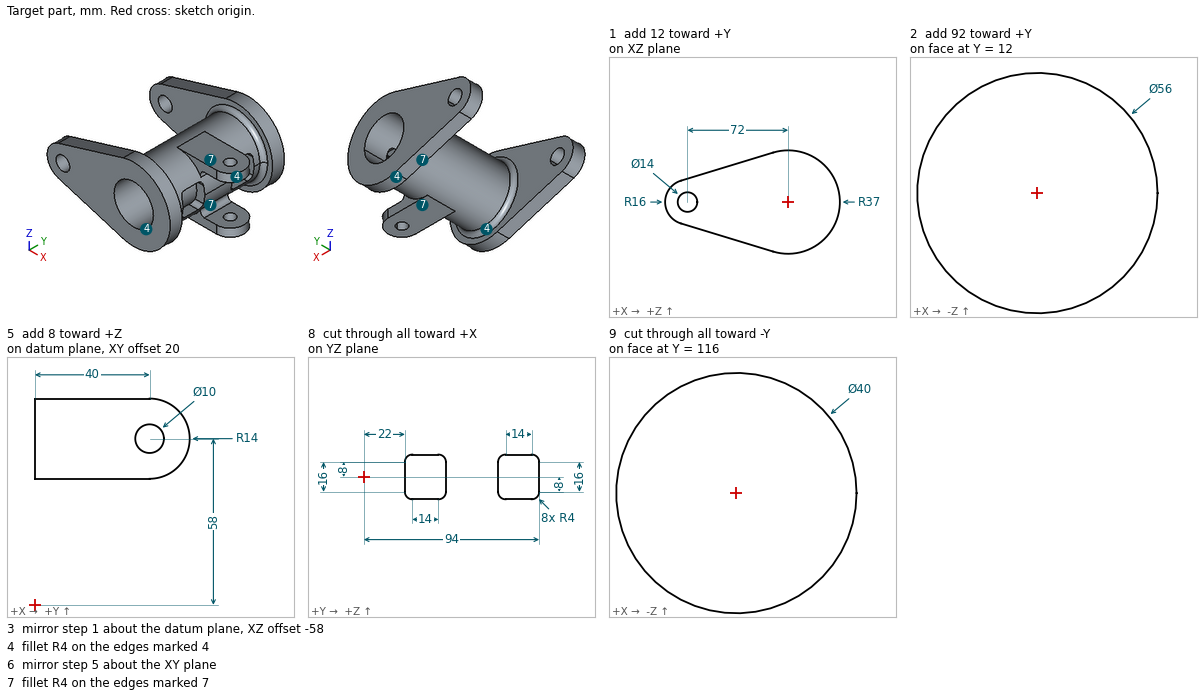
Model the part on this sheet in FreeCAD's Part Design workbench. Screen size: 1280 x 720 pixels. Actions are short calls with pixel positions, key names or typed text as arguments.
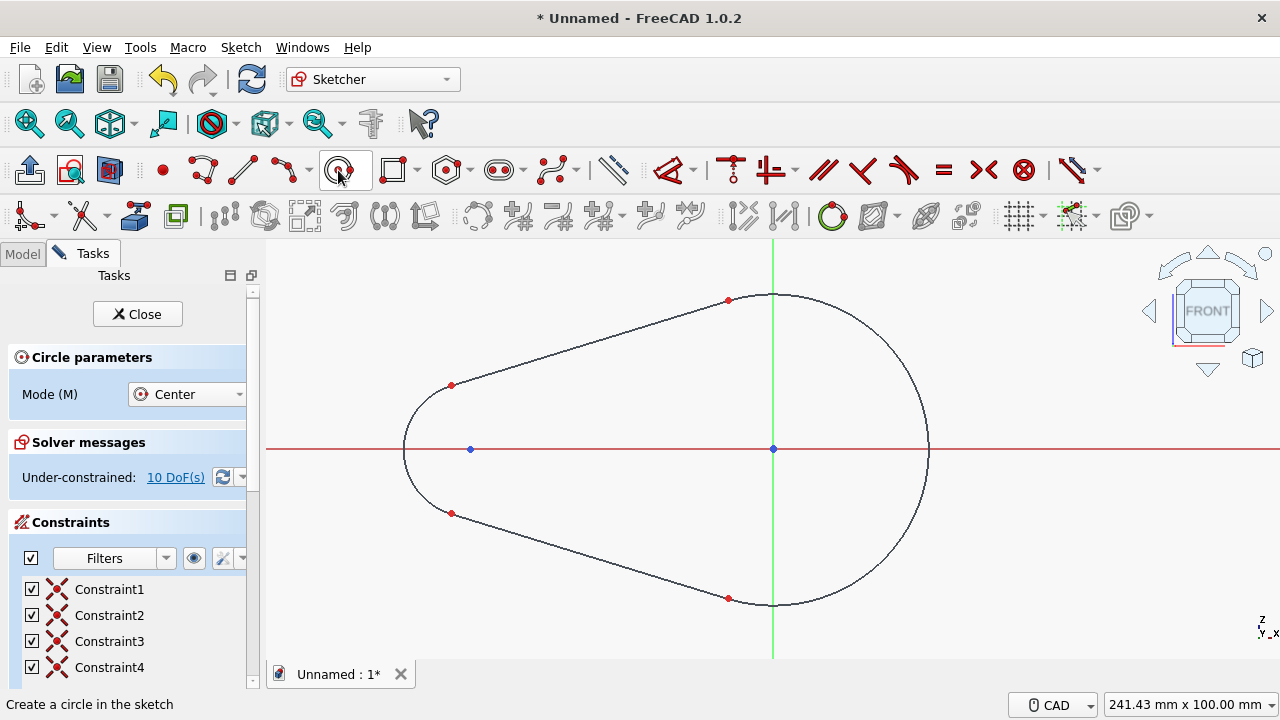
click(471, 449)
move(491, 428)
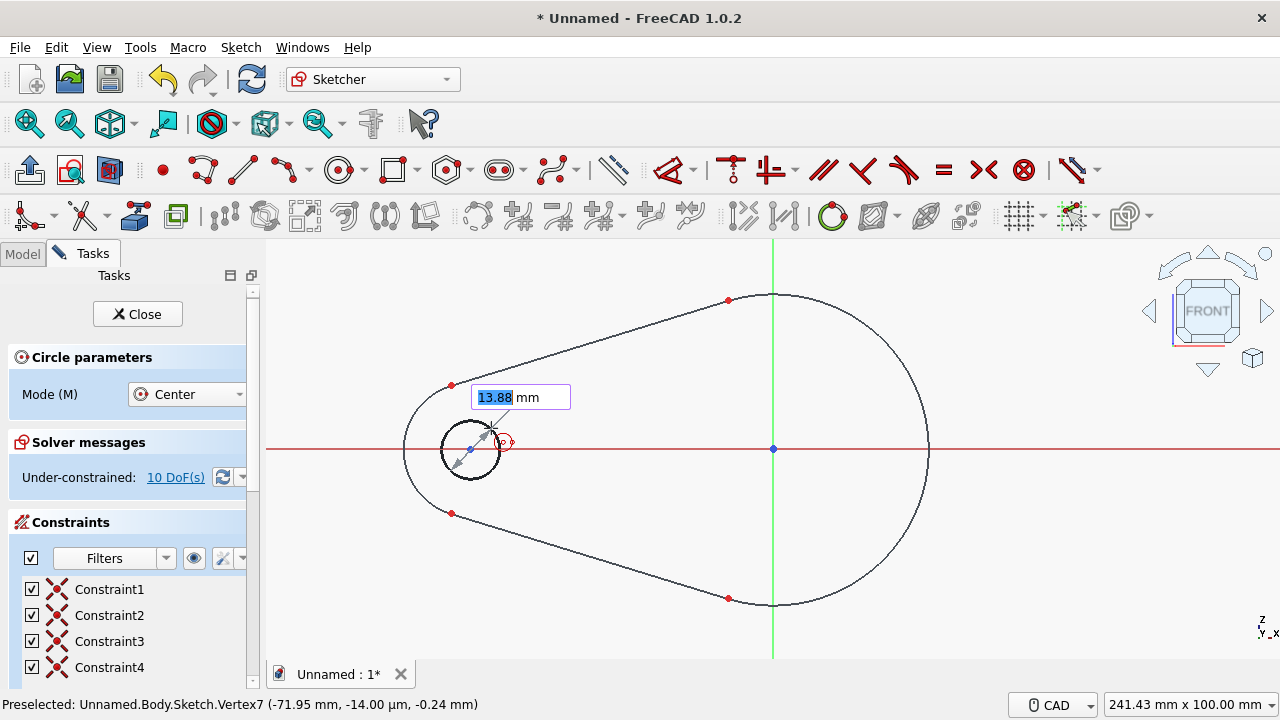
text(14)
key(Return)
key(Escape)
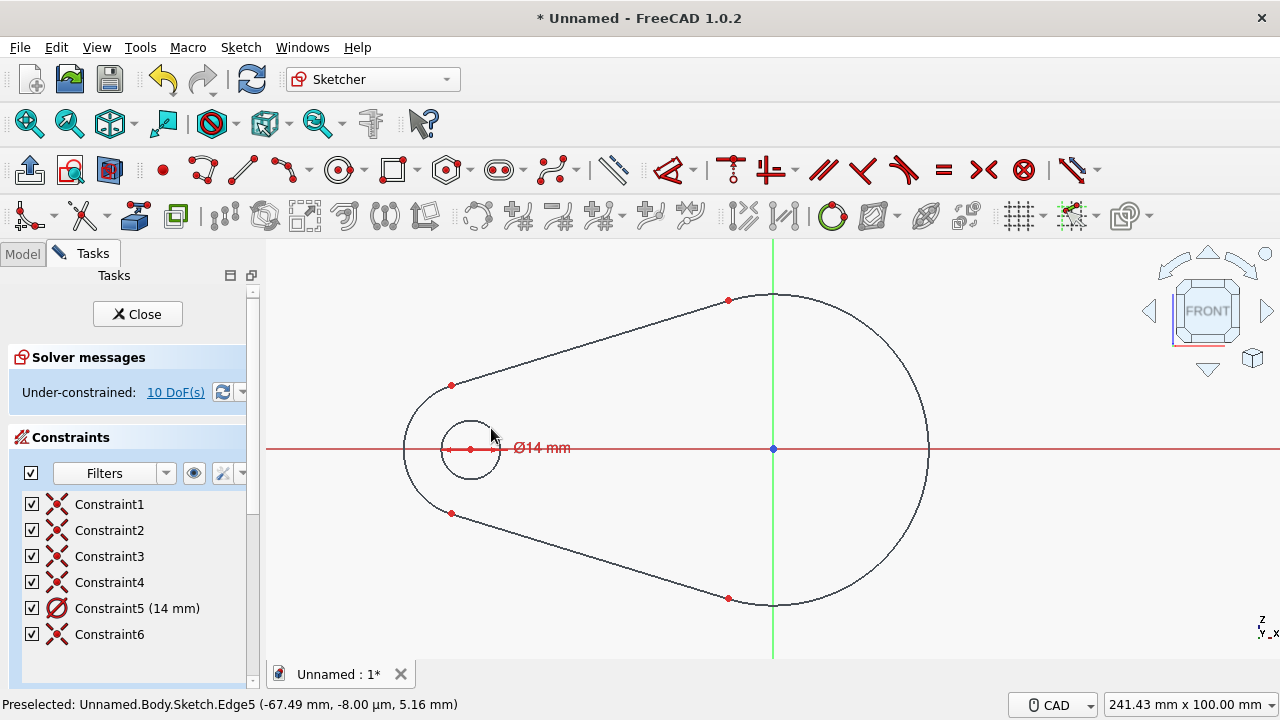
click(645, 574)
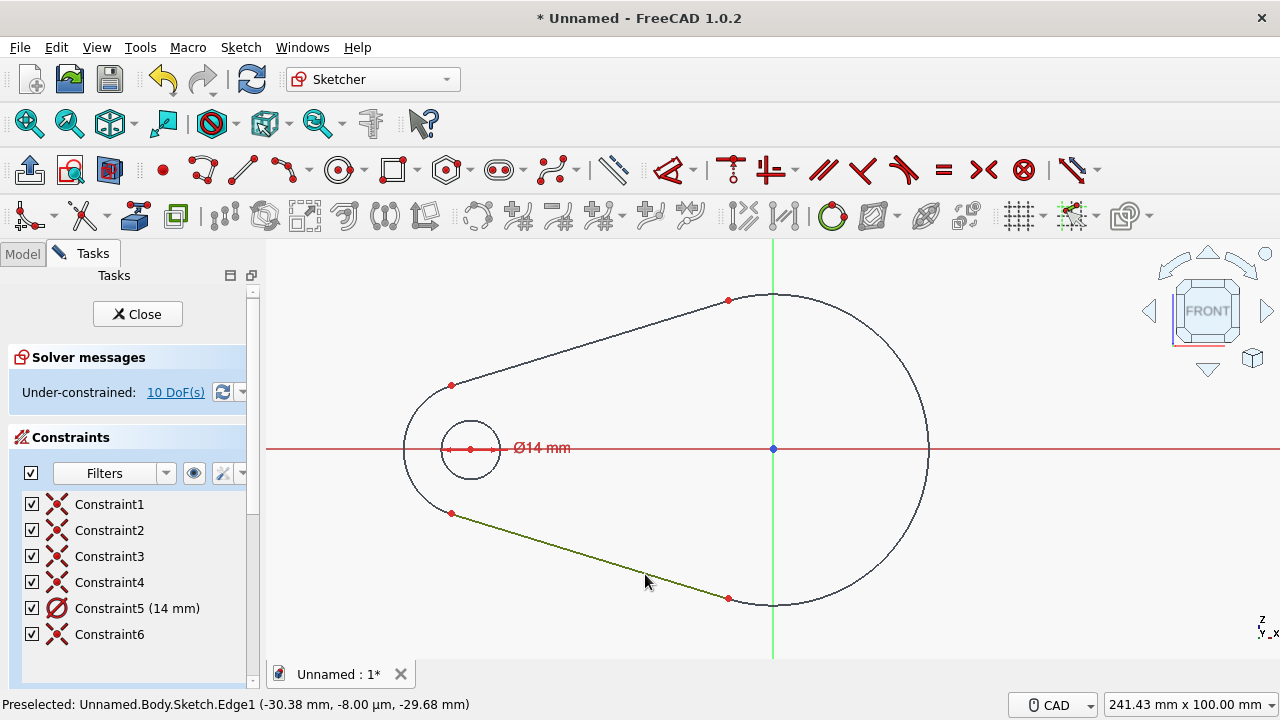
click(412, 417)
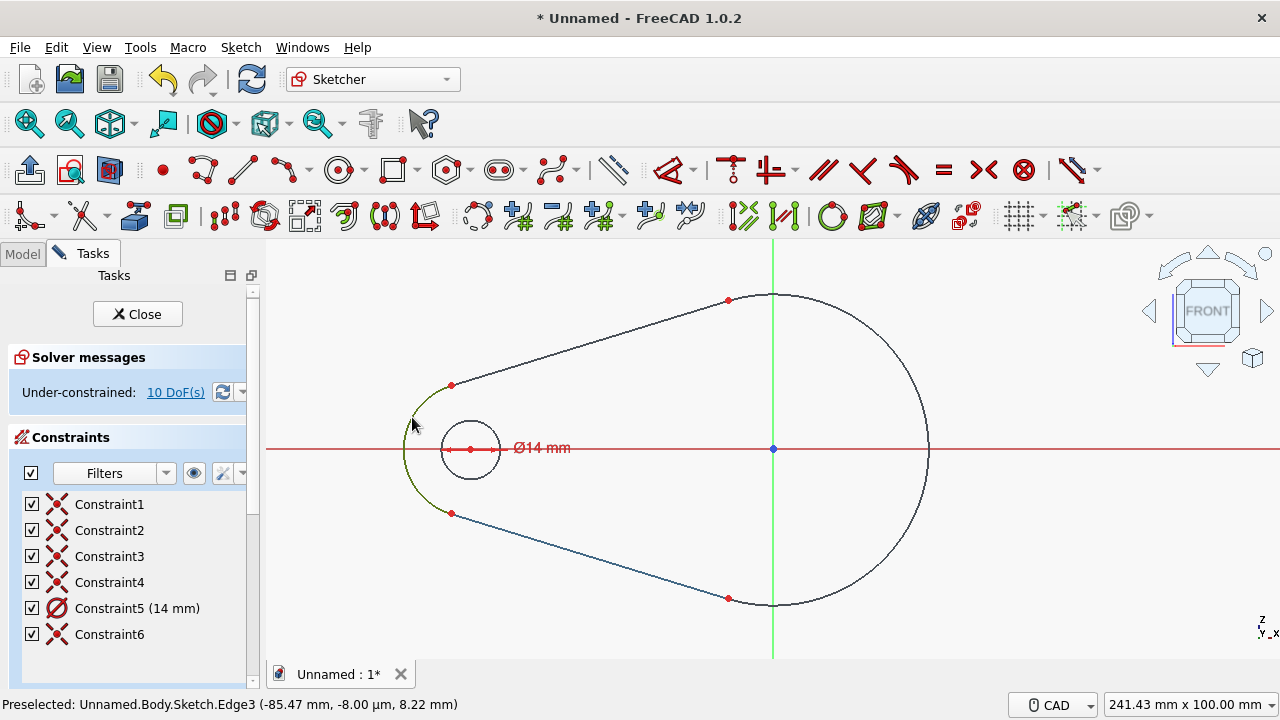
click(904, 170)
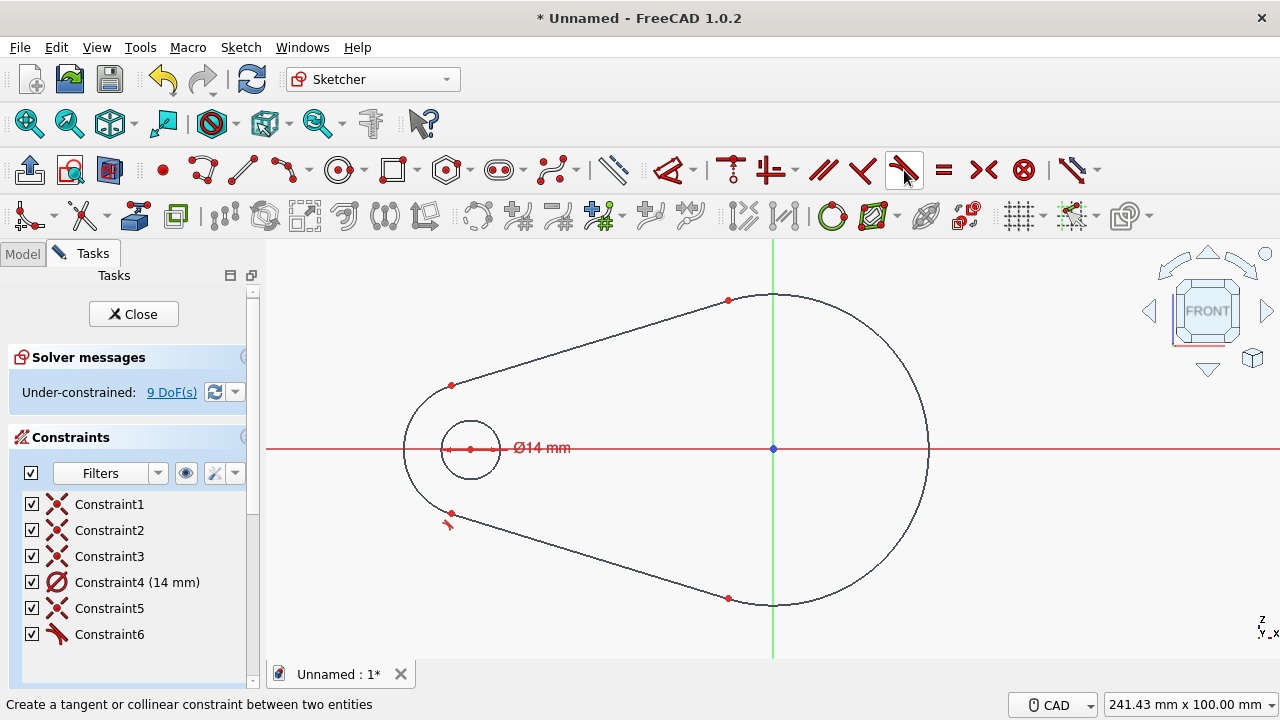
click(645, 574)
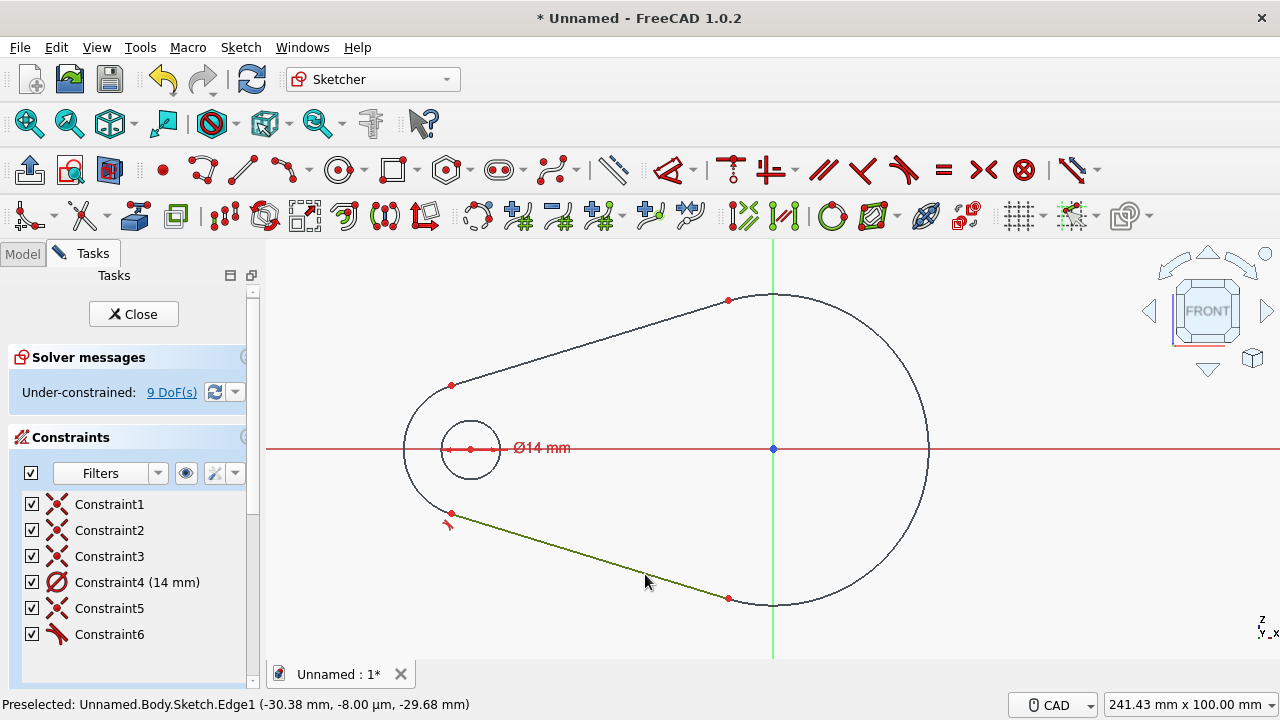
click(887, 556)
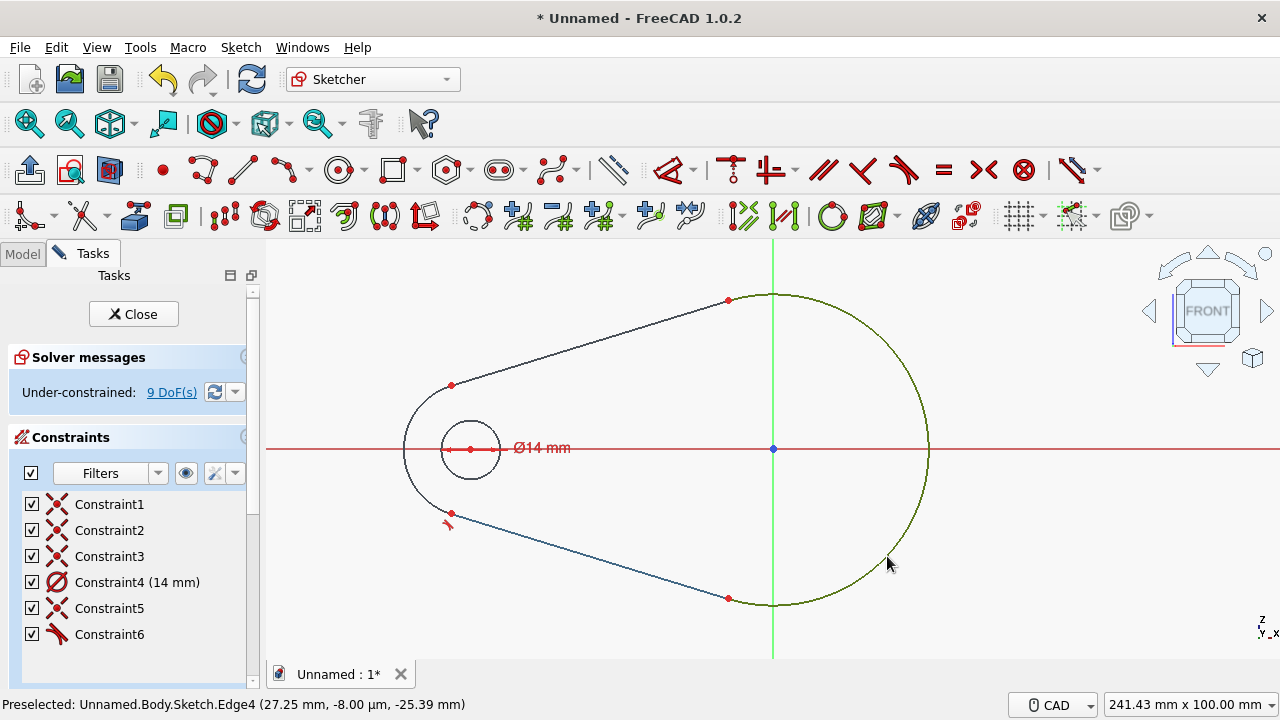
click(904, 170)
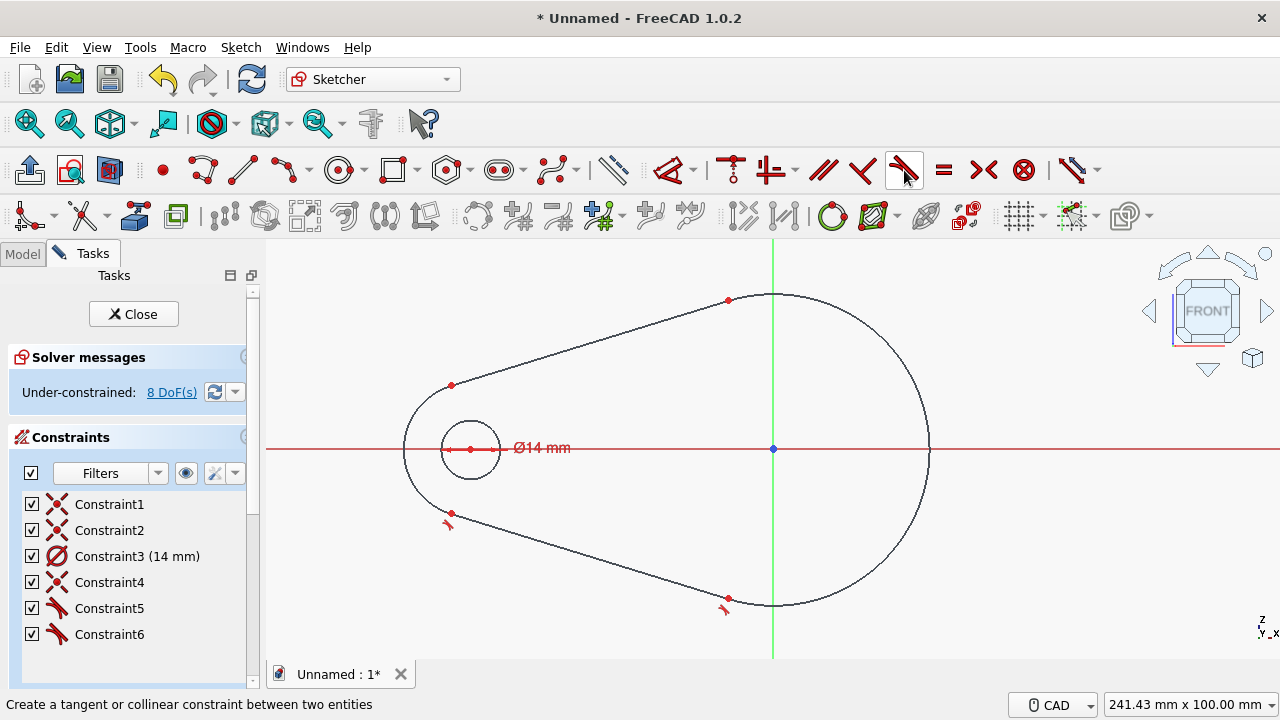
click(534, 361)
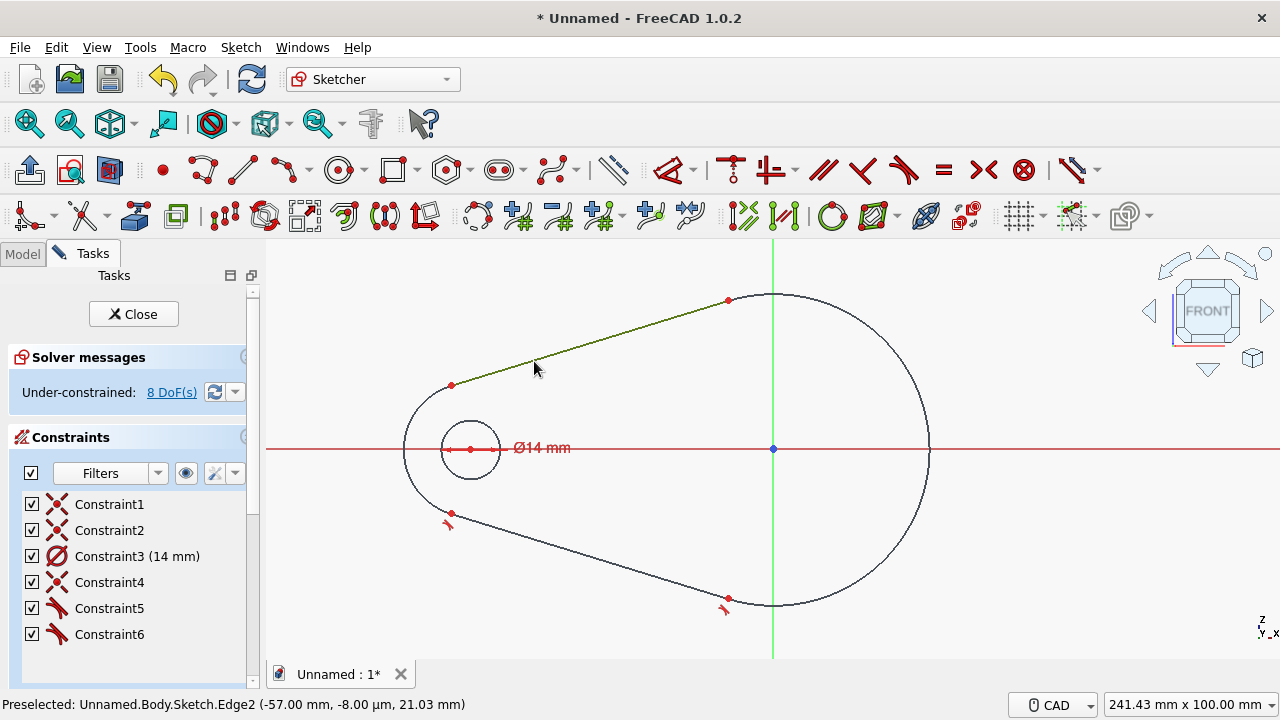
click(412, 417)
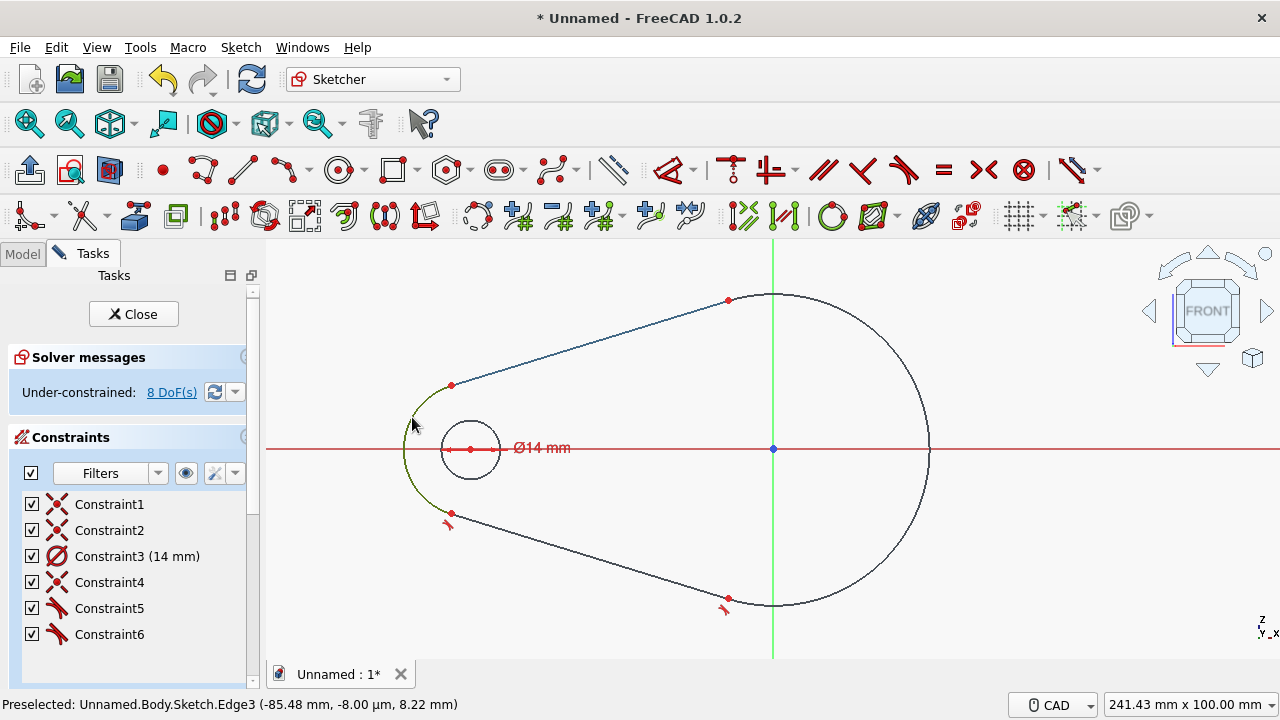
click(904, 170)